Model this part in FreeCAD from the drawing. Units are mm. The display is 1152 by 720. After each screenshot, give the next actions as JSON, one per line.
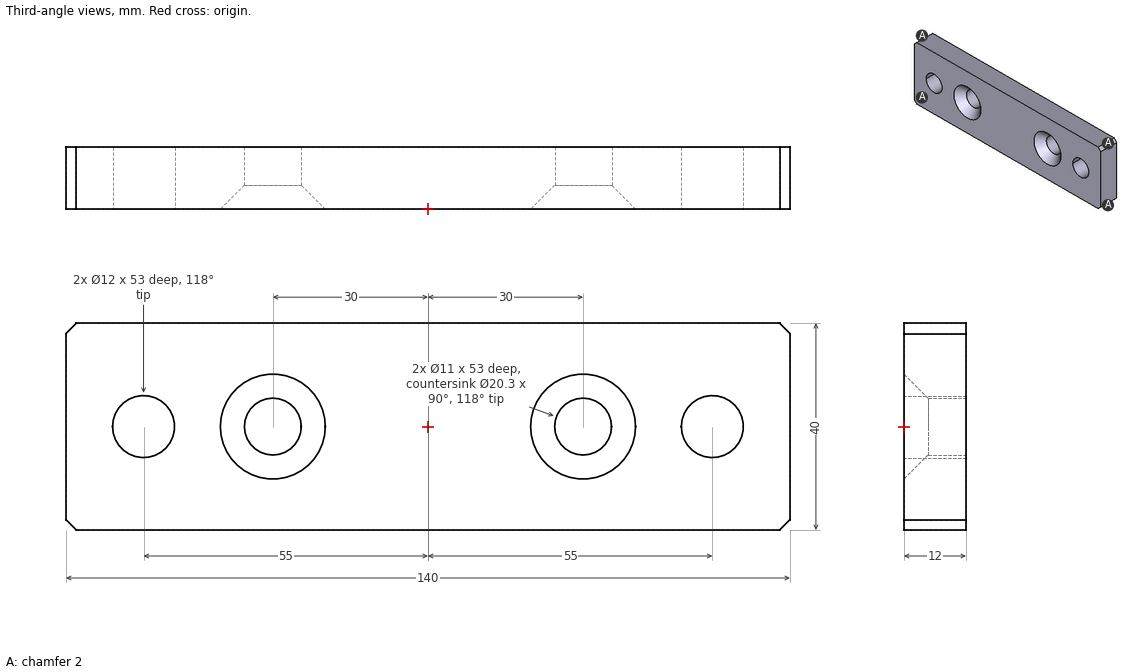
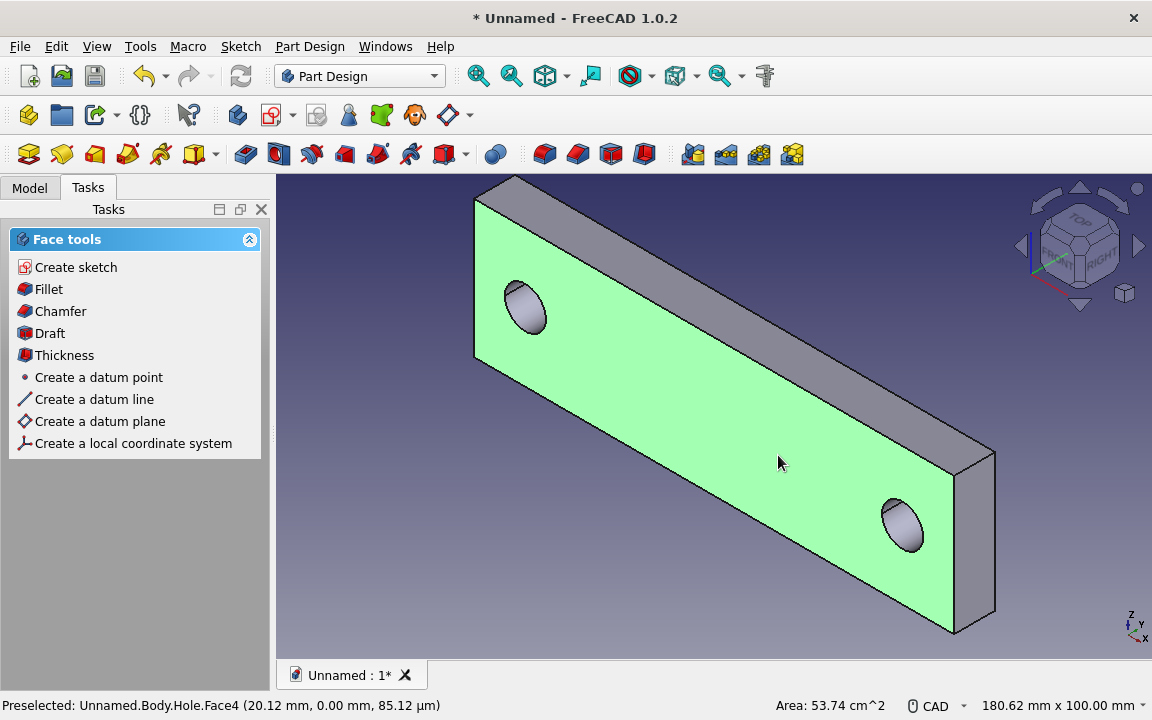
{"action": "left_click", "coordinate": [270, 116]}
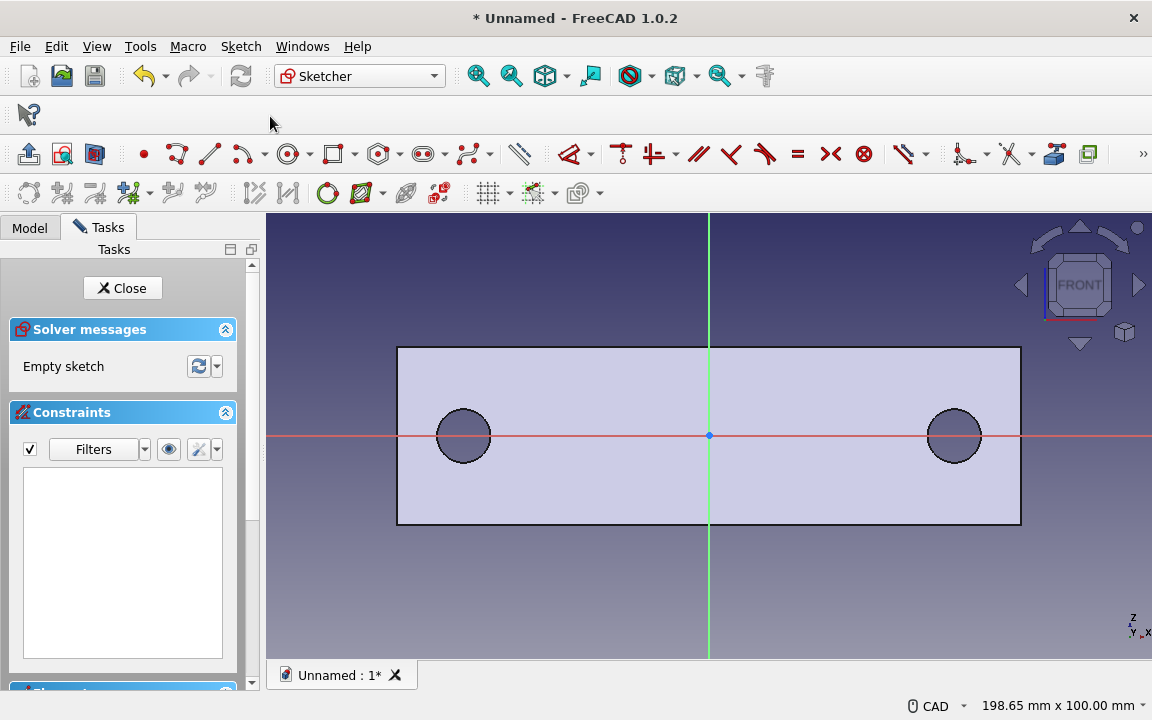
{"action": "scroll", "coordinate": [848, 436], "scroll_direction": "up", "scroll_amount": 2}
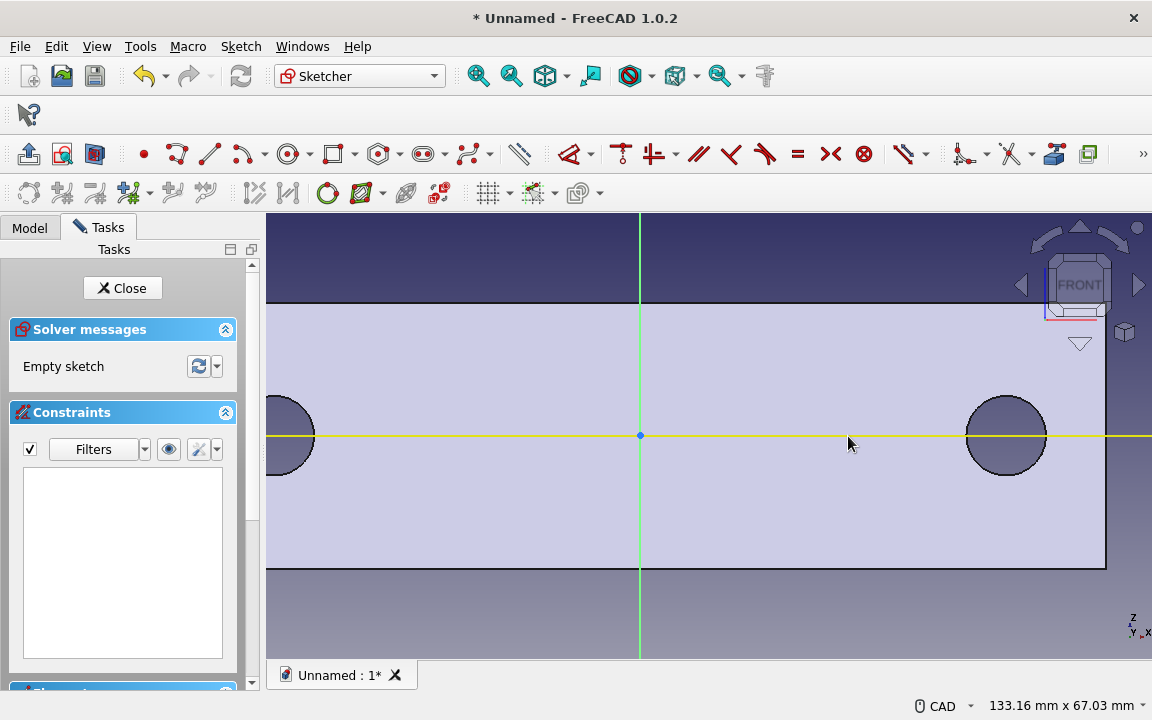
{"action": "key", "text": "g c"}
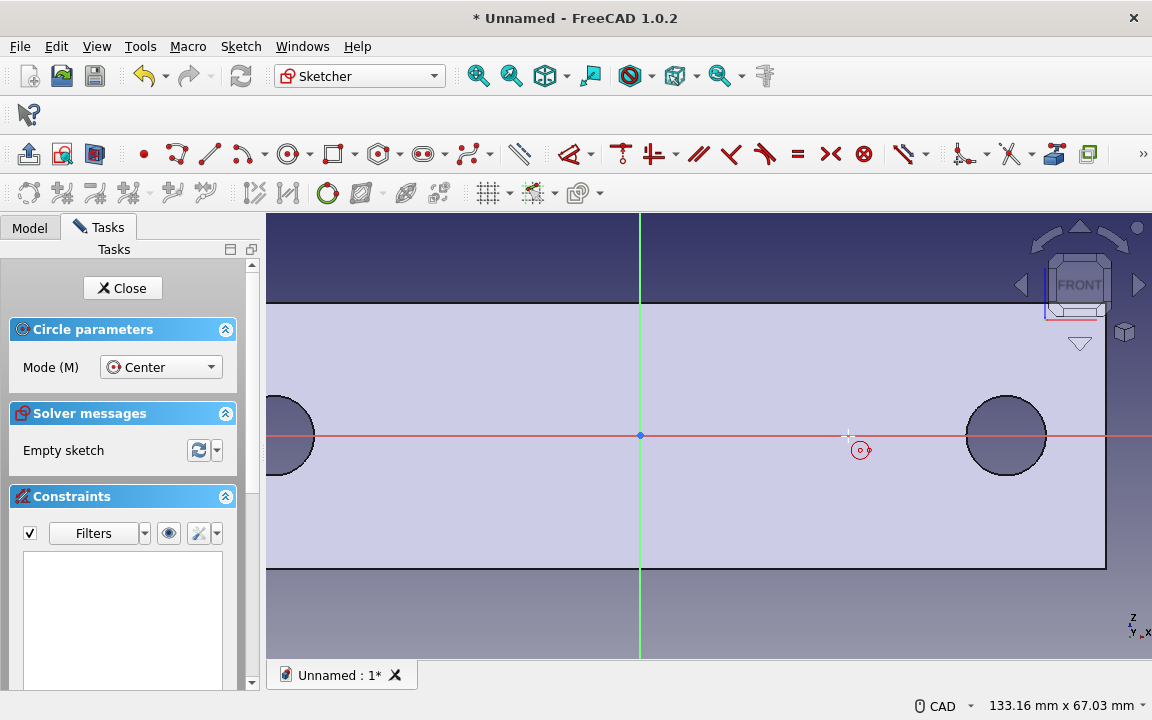
{"action": "left_click", "coordinate": [840, 436]}
{"action": "mouse_move", "coordinate": [866, 410]}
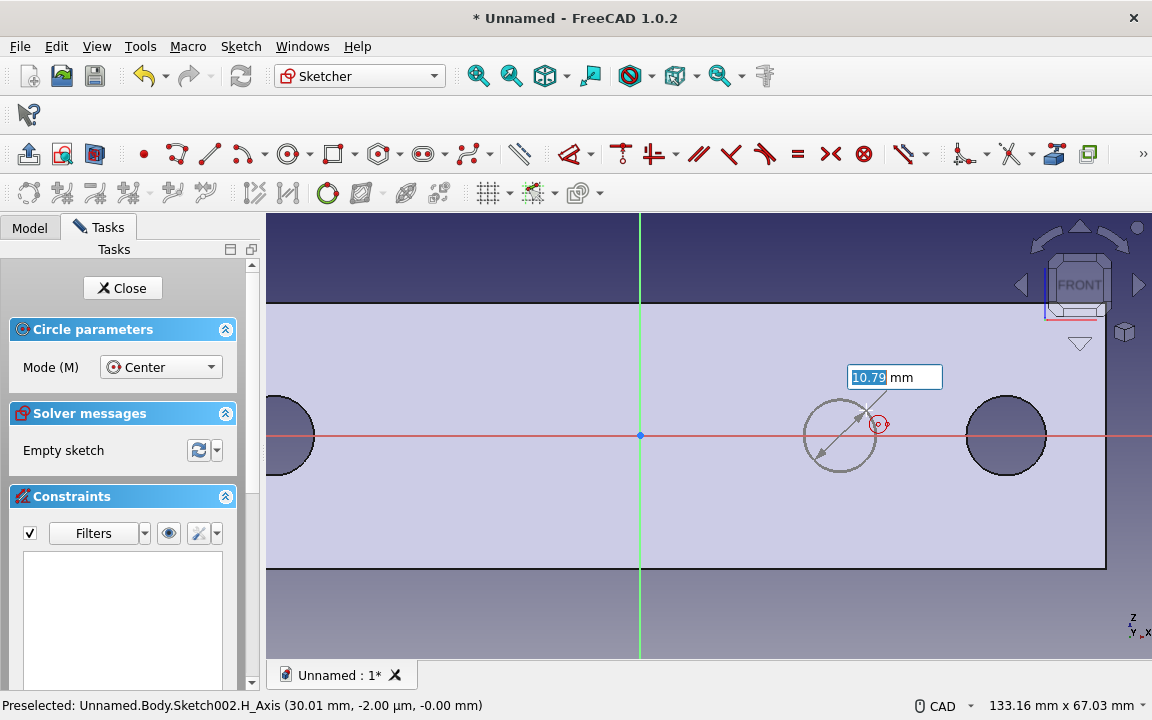
{"action": "type", "text": "11"}
{"action": "key", "text": "Return"}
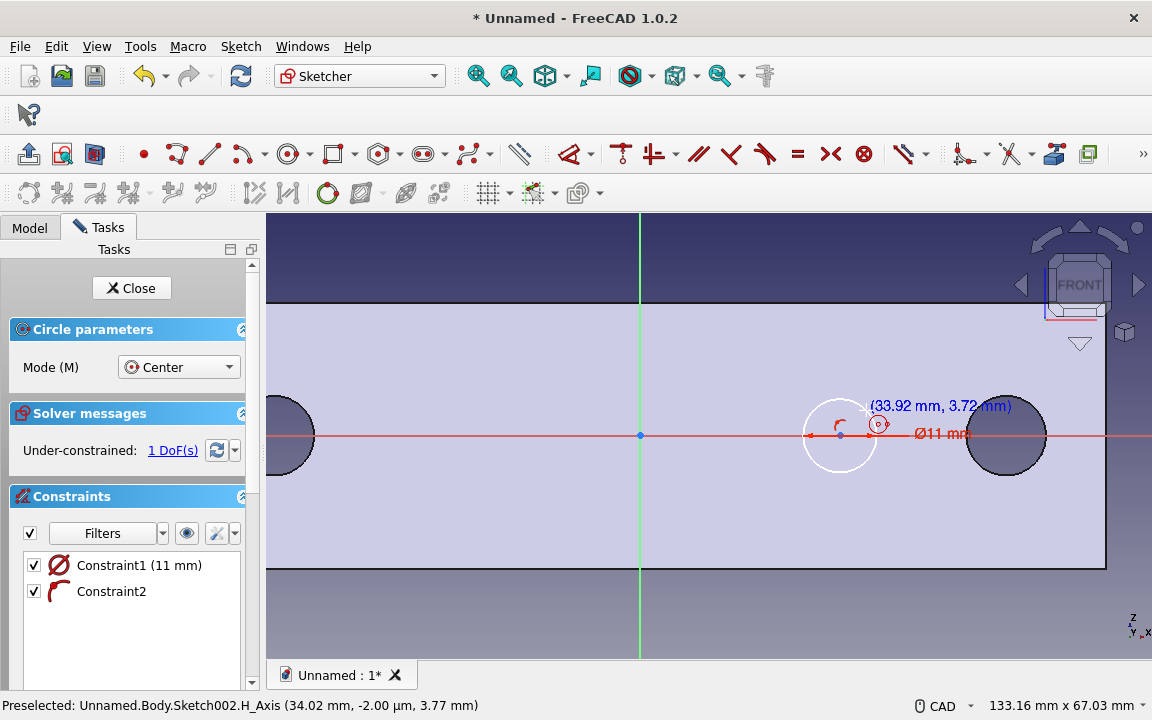
{"action": "left_click", "coordinate": [441, 436]}
{"action": "mouse_move", "coordinate": [467, 410]}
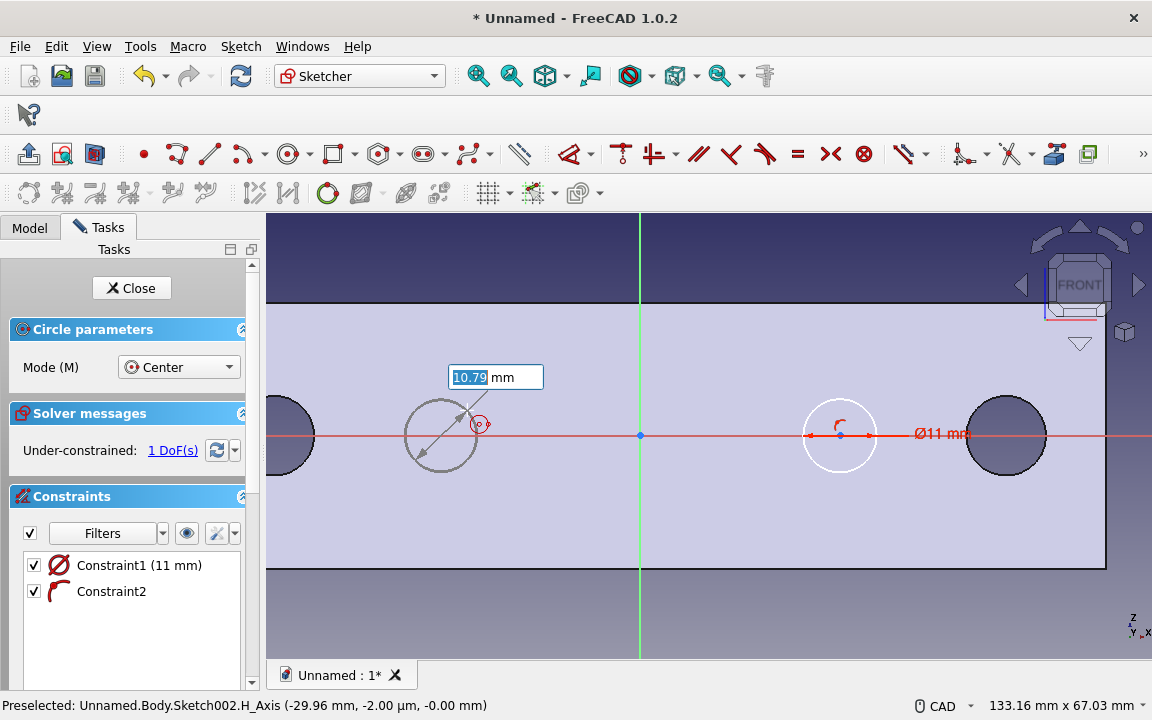
{"action": "type", "text": "11"}
{"action": "key", "text": "Return"}
{"action": "key", "text": "Escape"}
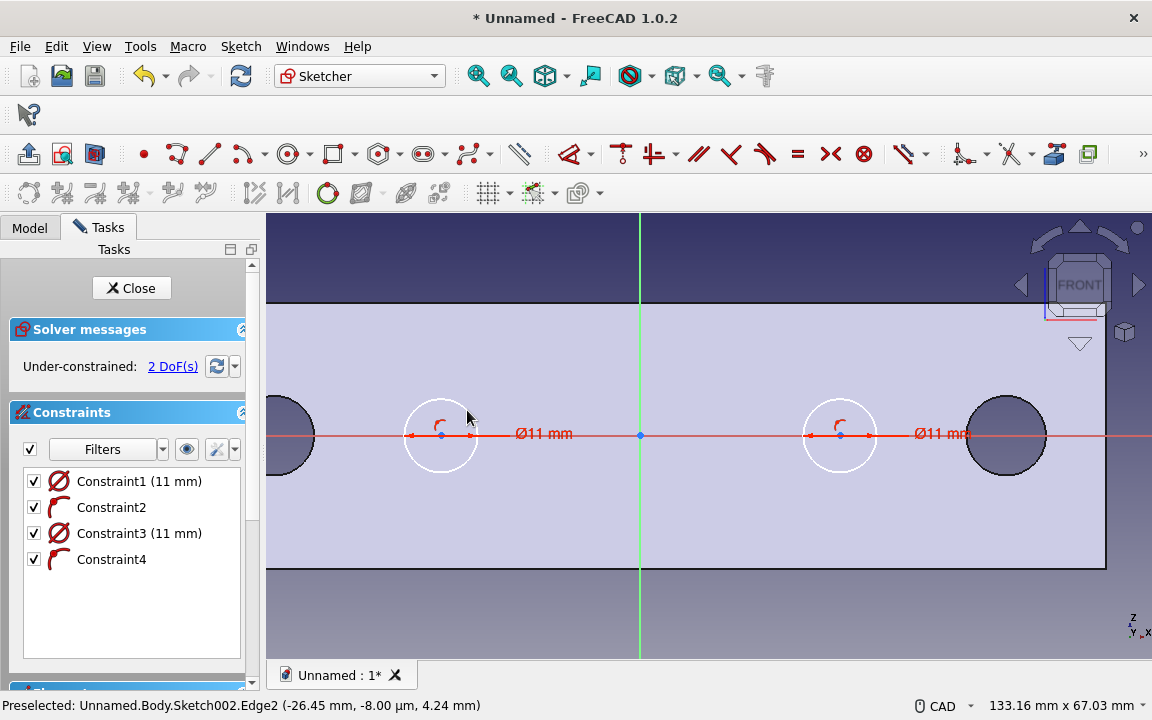
{"action": "left_click", "coordinate": [568, 154]}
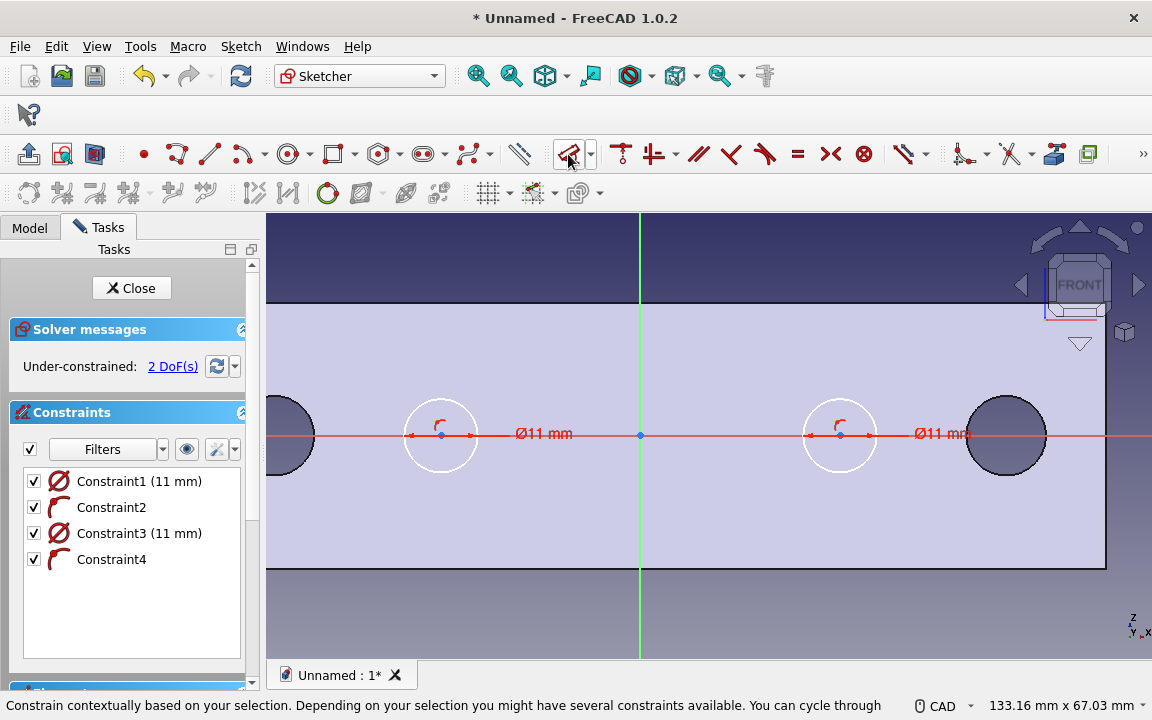
{"action": "left_click", "coordinate": [840, 436]}
{"action": "left_click", "coordinate": [740, 470]}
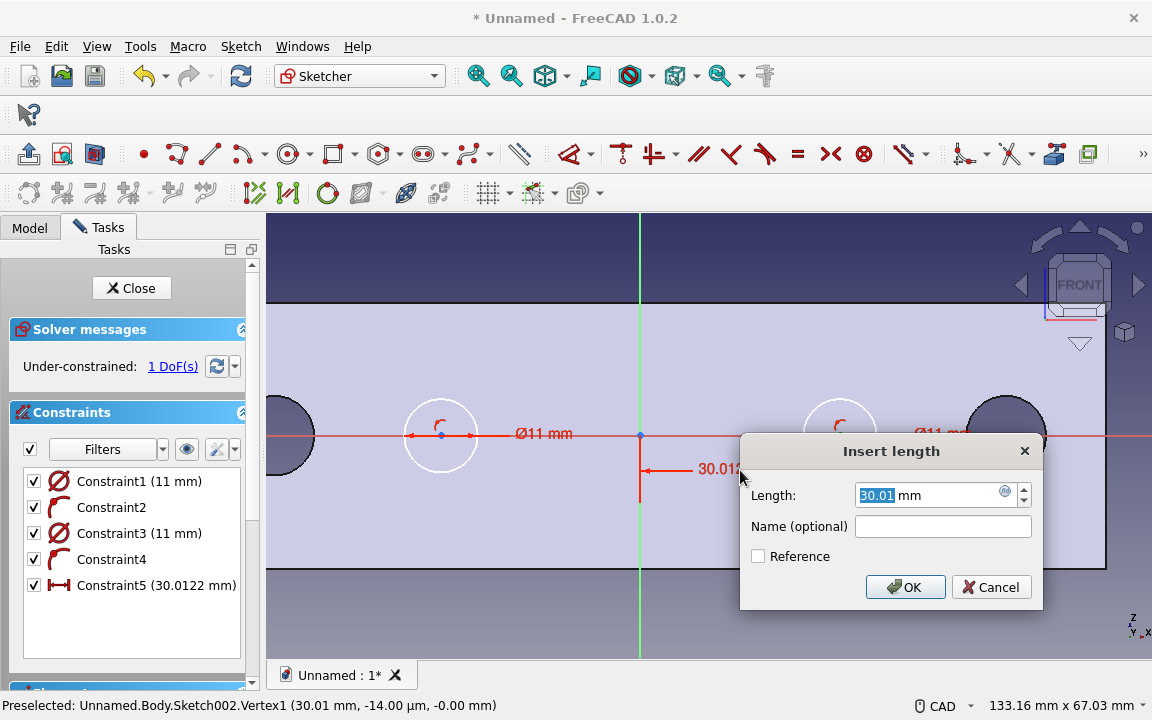
{"action": "type", "text": "30"}
{"action": "key", "text": "Return"}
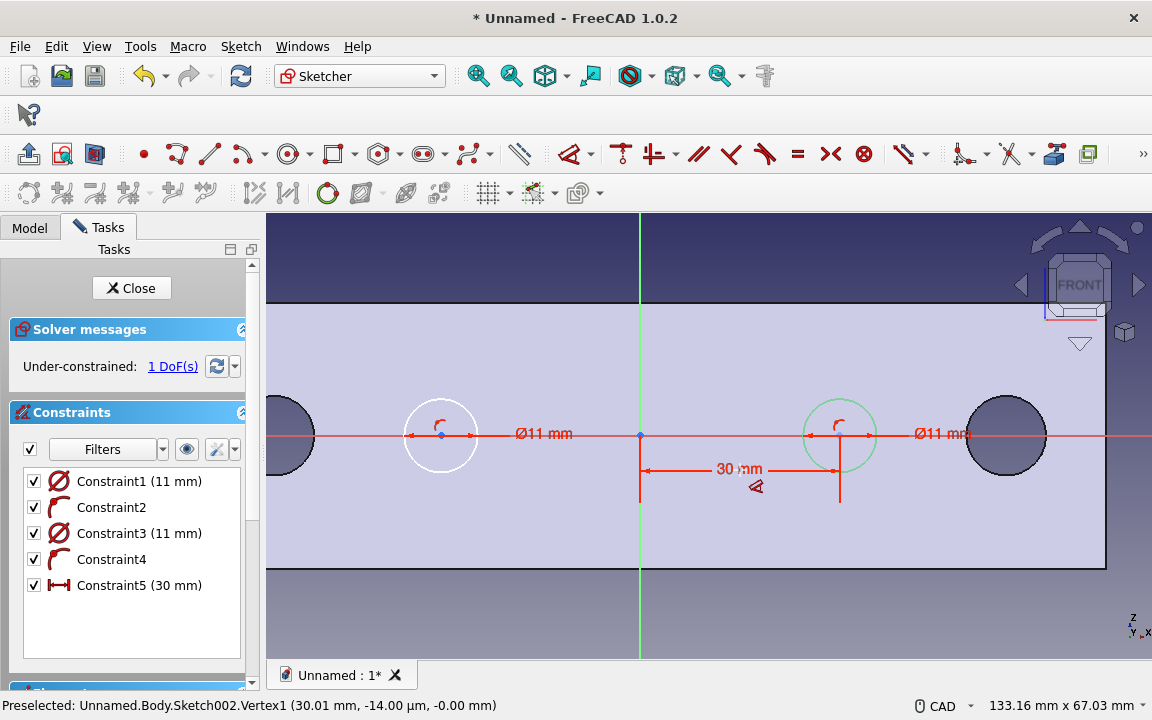
{"action": "left_click", "coordinate": [441, 436]}
{"action": "left_click", "coordinate": [541, 470]}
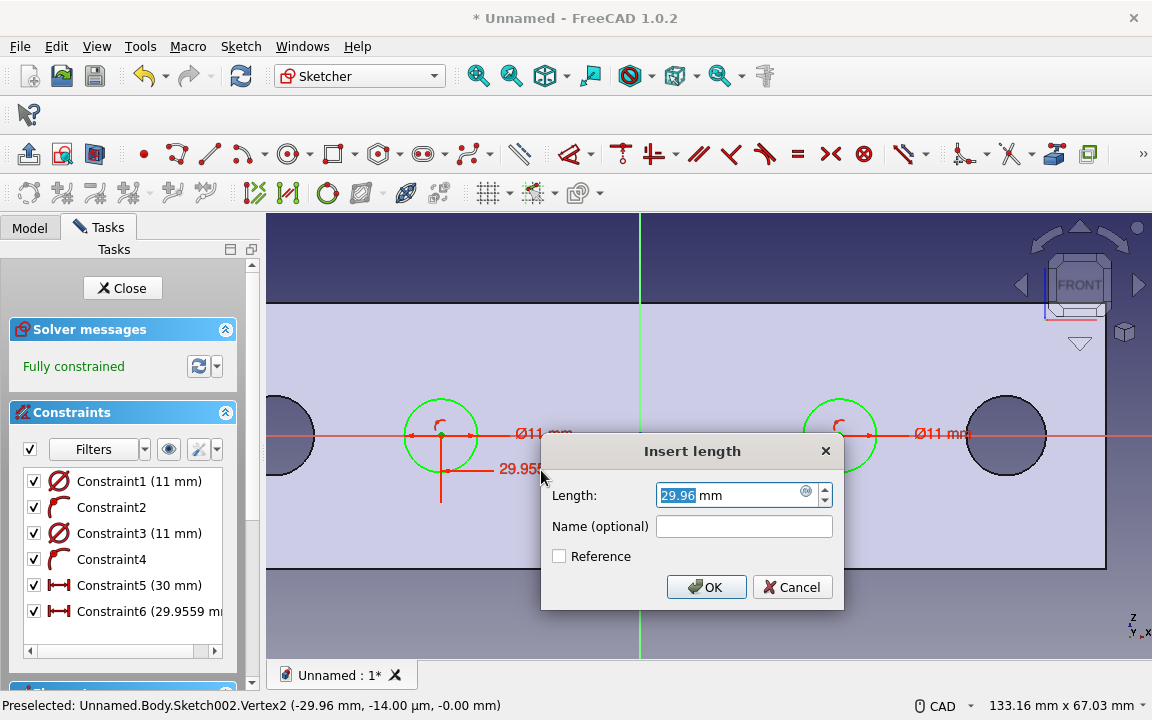
{"action": "type", "text": "30"}
{"action": "key", "text": "Return"}
{"action": "key", "text": "Escape"}